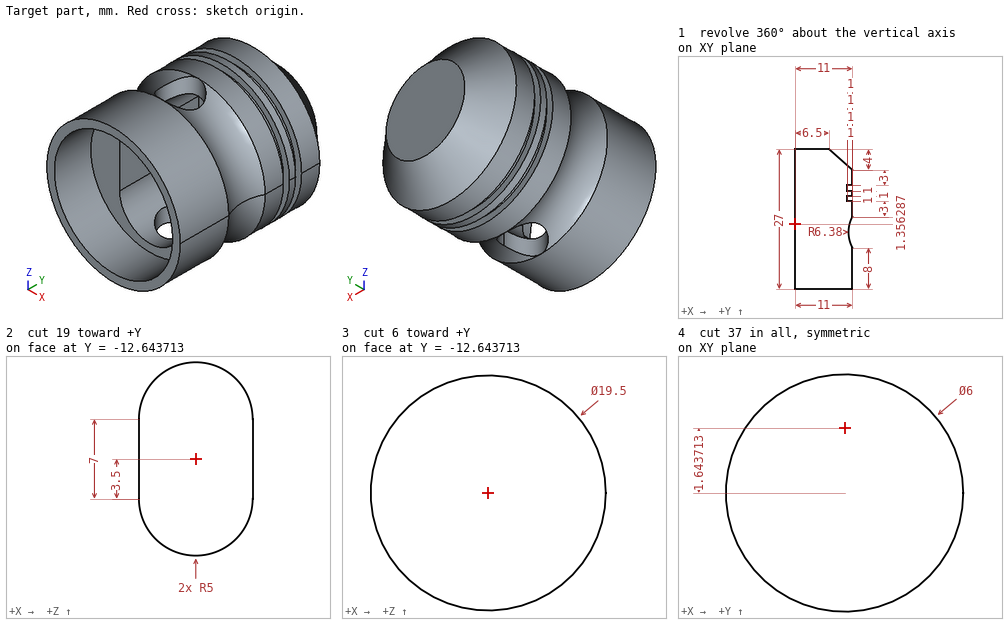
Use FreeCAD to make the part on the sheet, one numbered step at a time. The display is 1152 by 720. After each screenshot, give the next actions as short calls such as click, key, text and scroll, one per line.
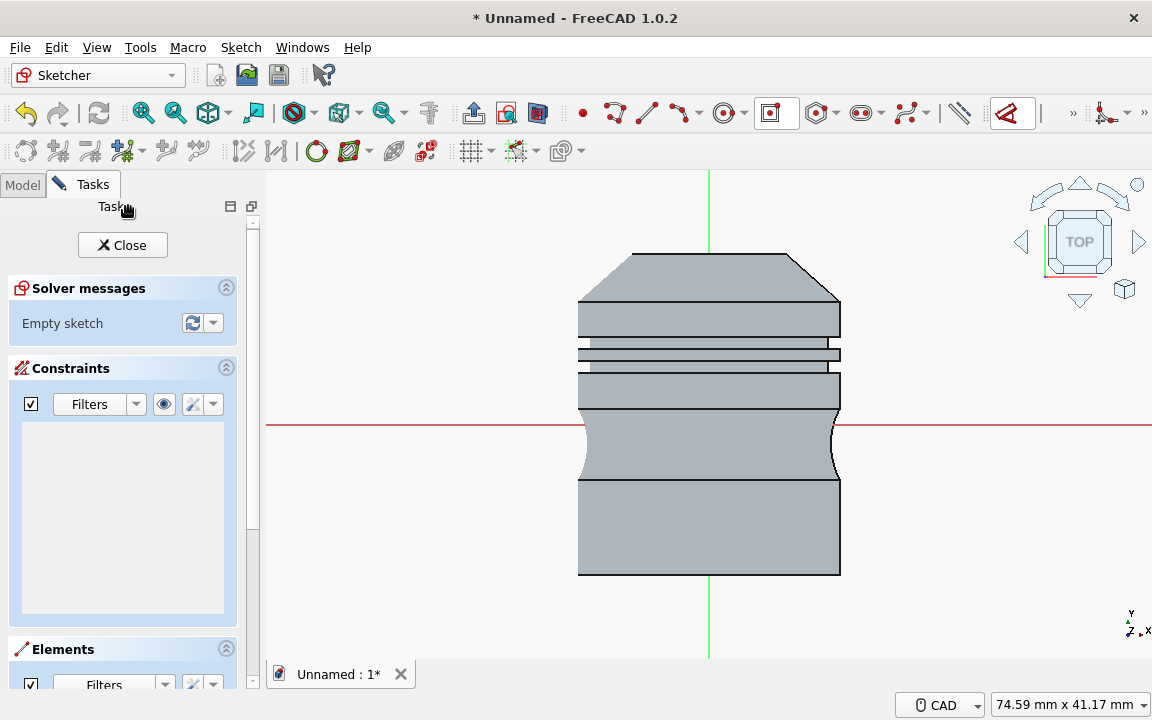
click(538, 114)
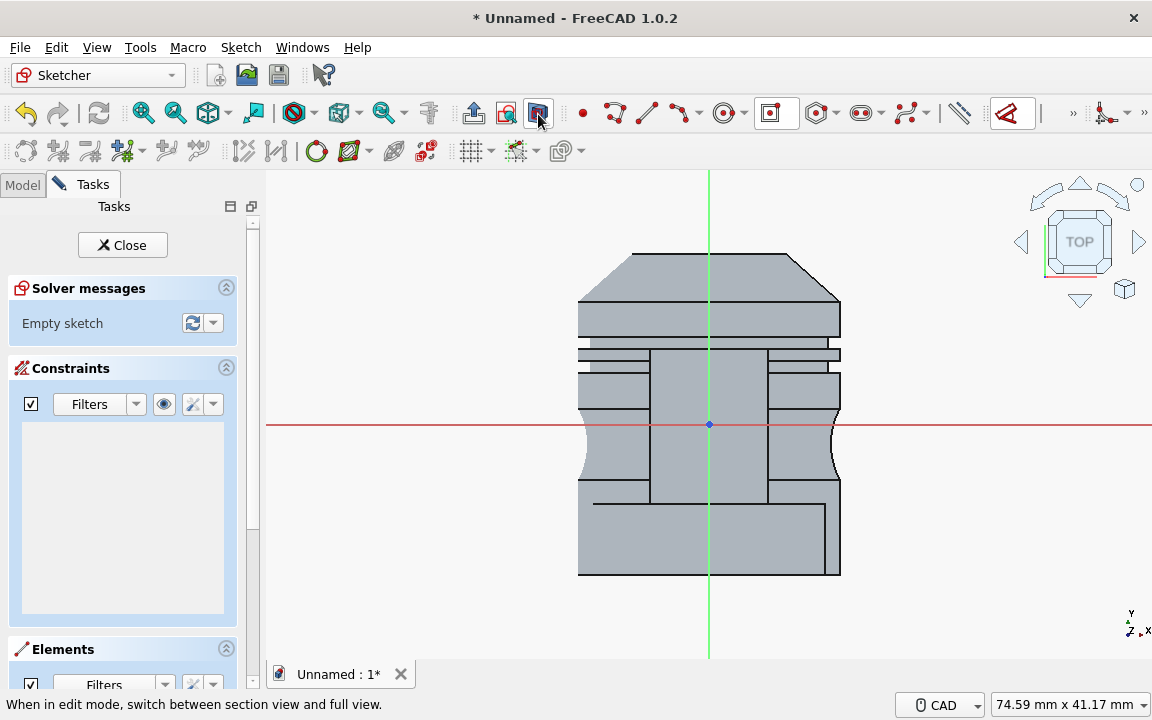
scroll(731, 454, up, 7)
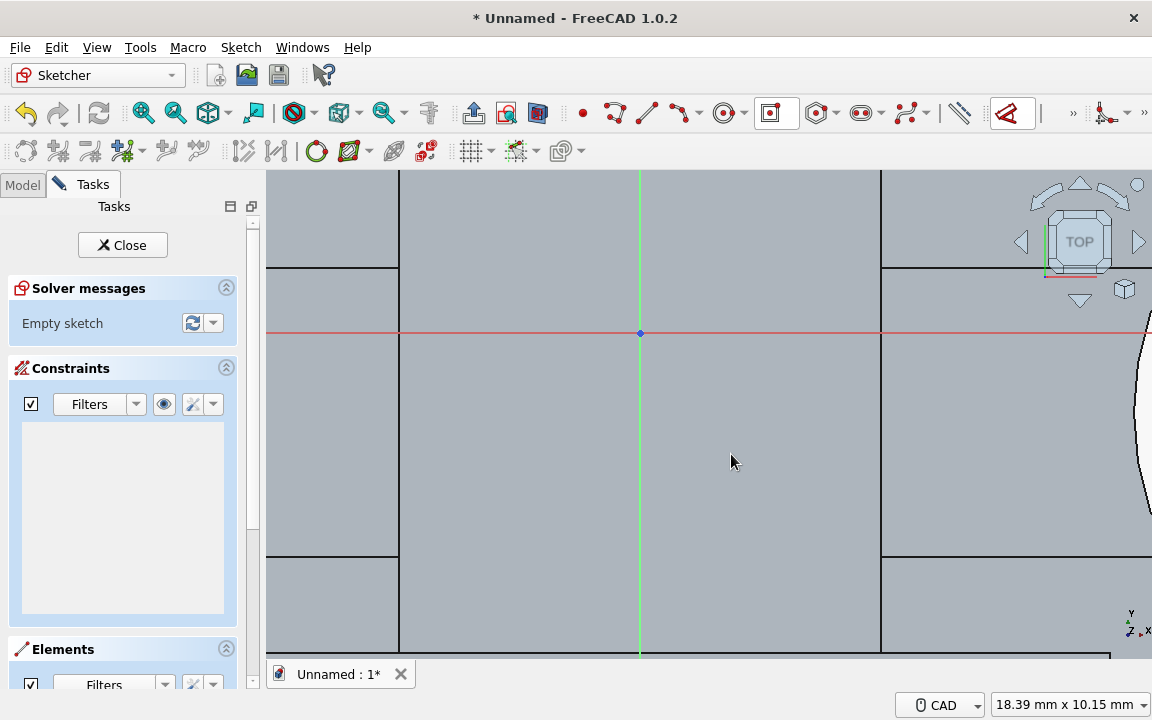
click(724, 114)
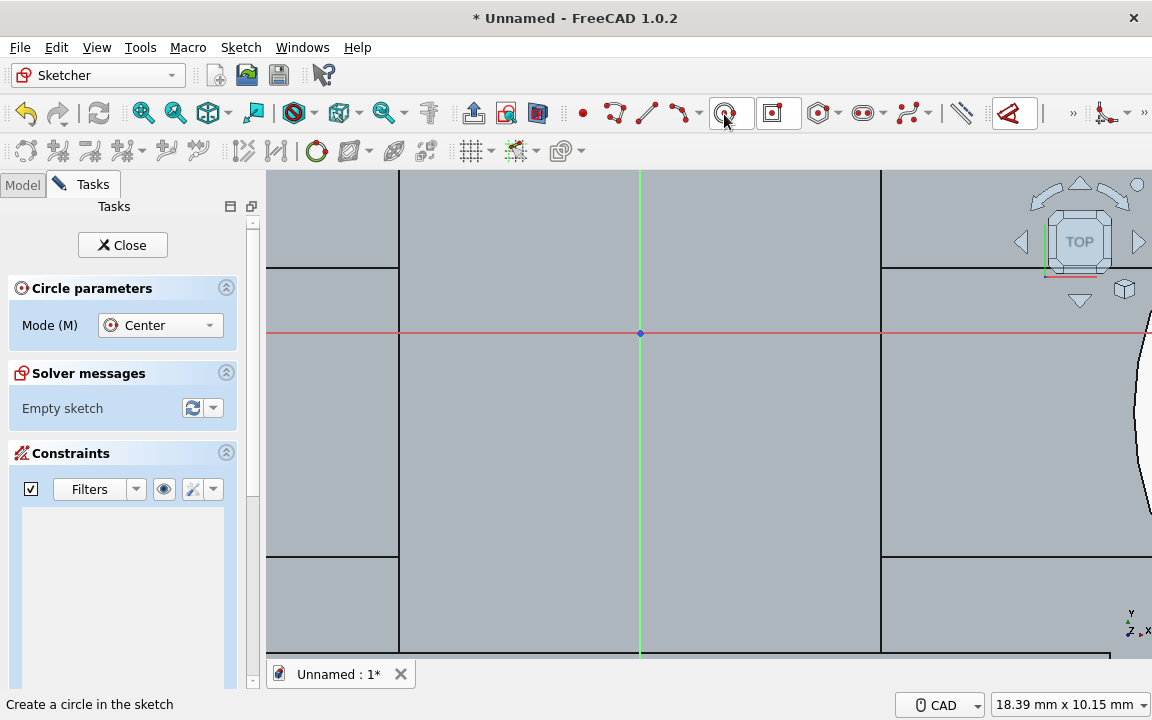
click(640, 412)
move(742, 310)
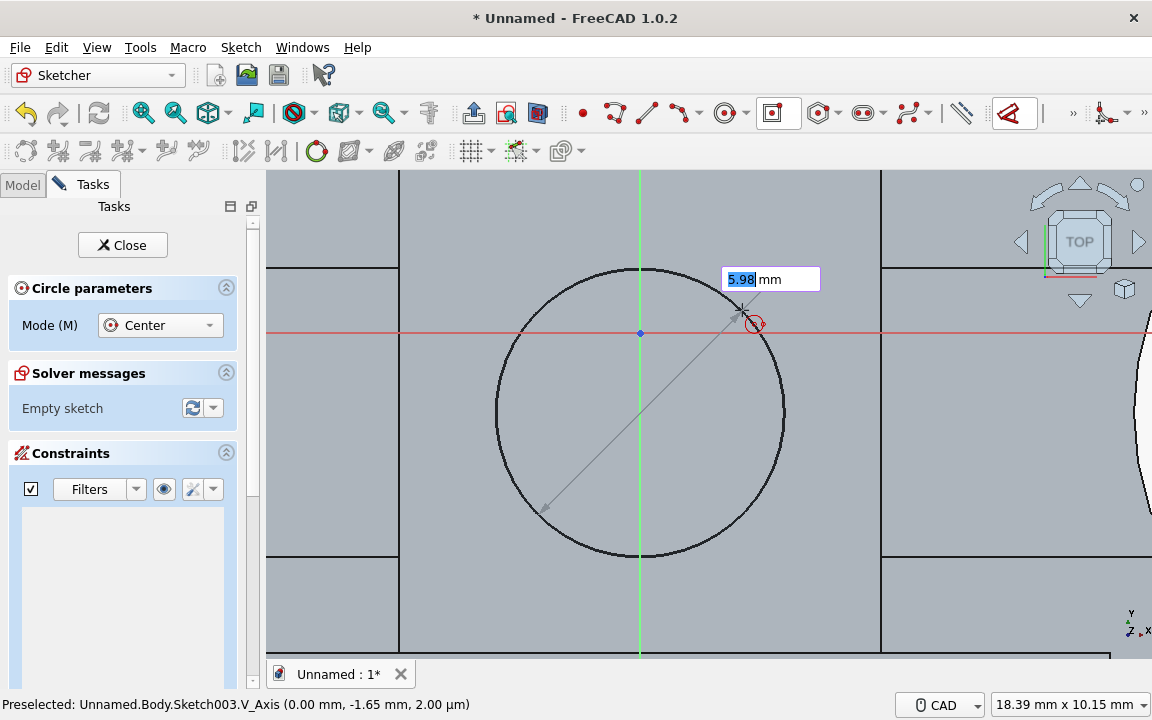
text(6)
key(Return)
key(Escape)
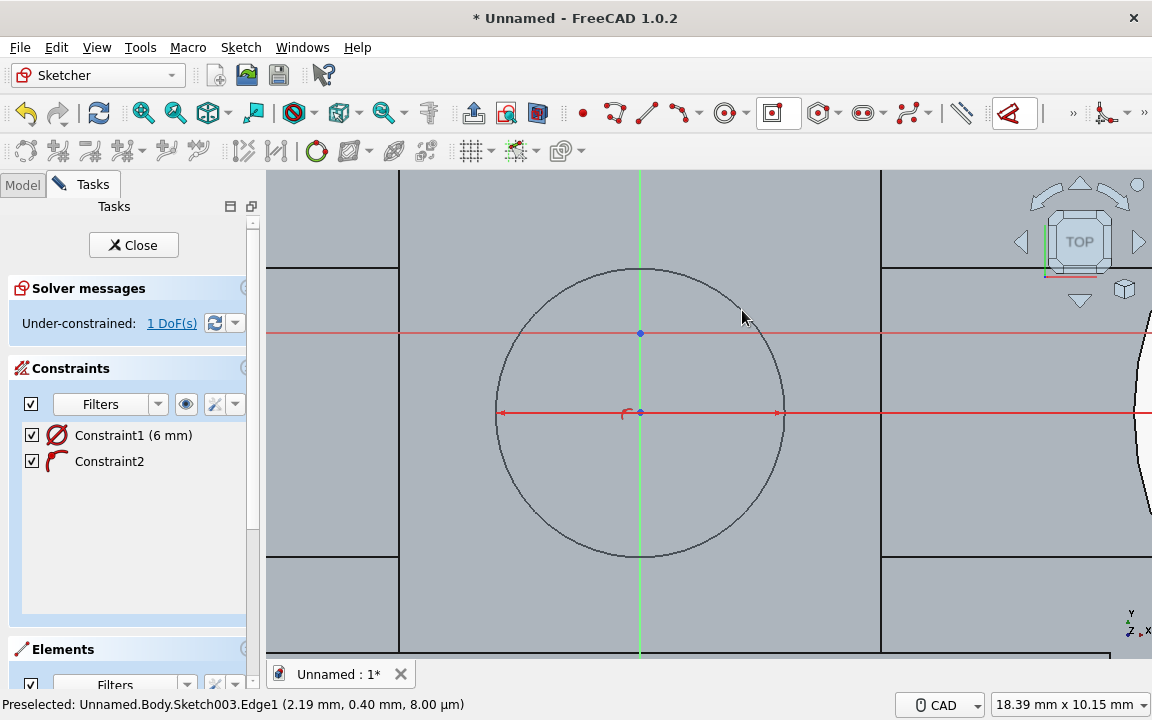
click(640, 413)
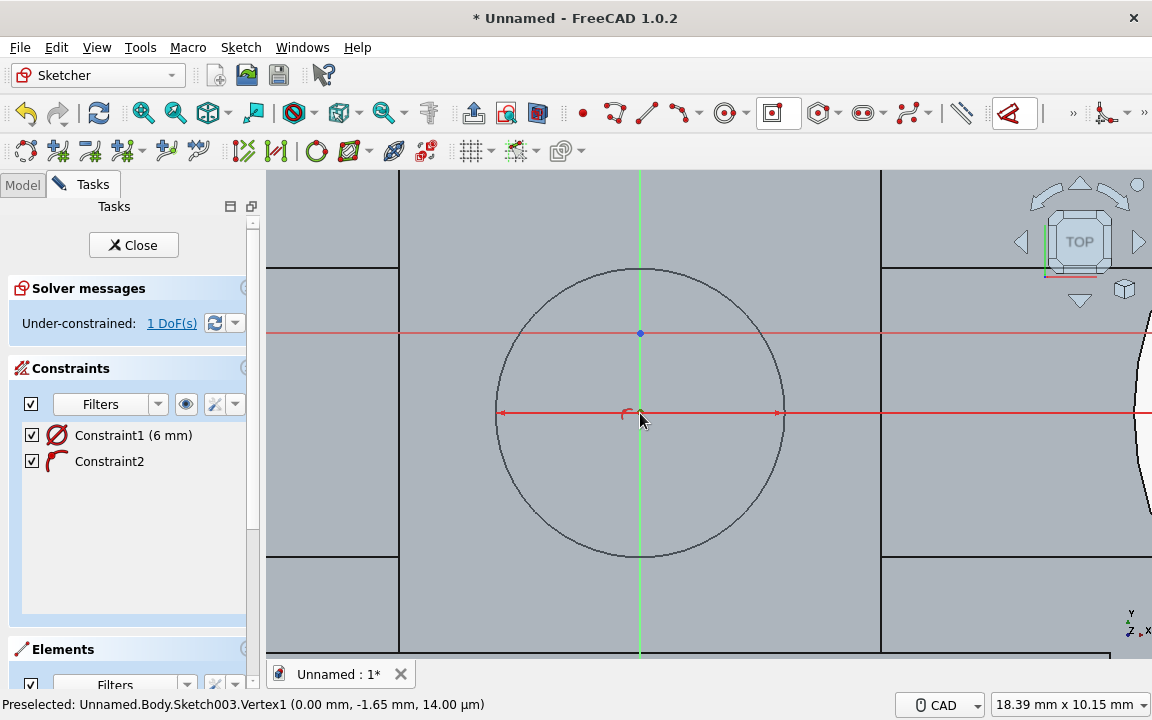
click(1032, 114)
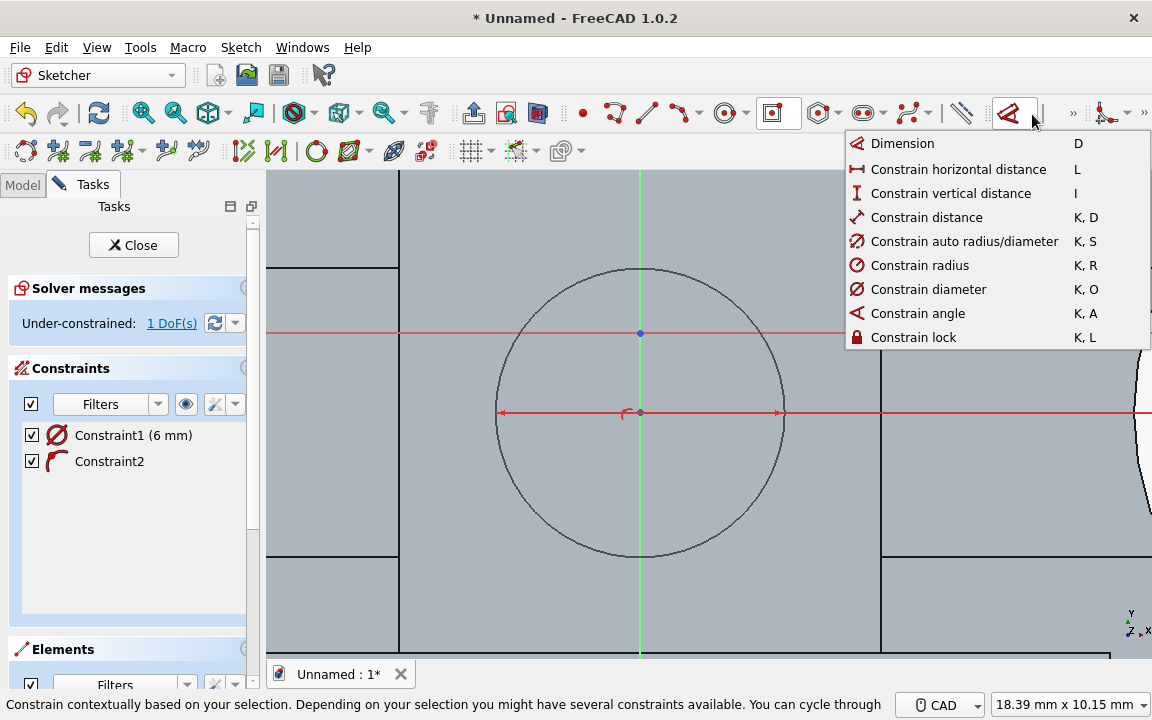
click(998, 193)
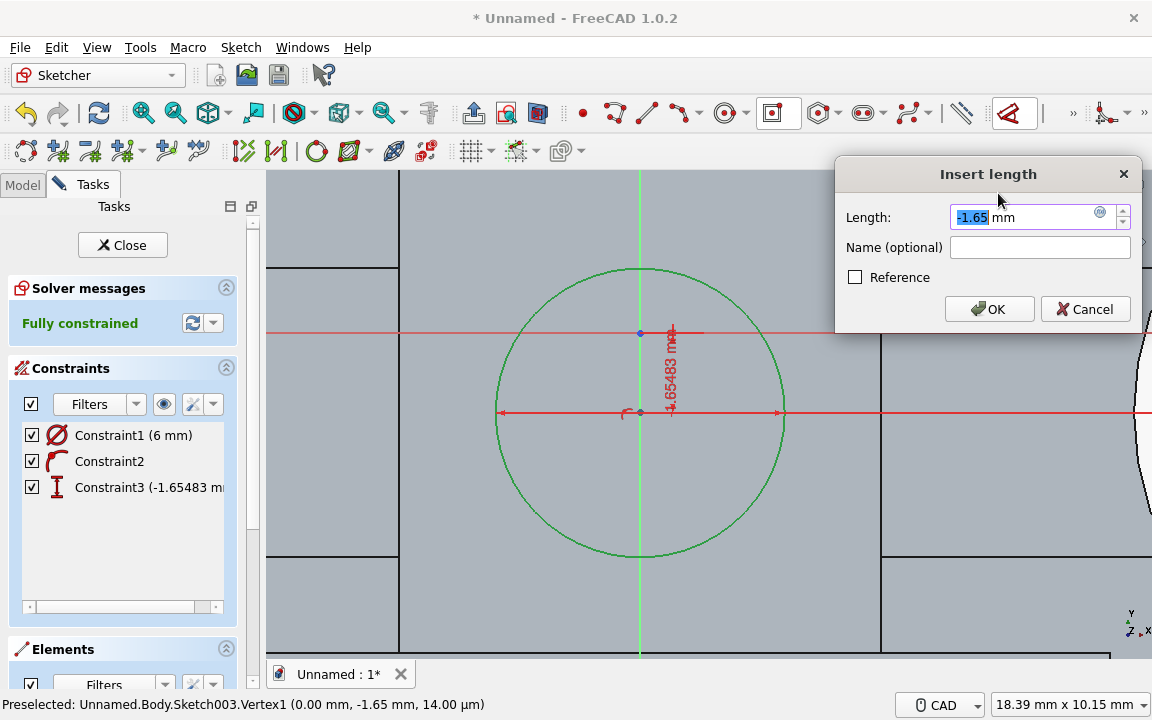
text(-1.643713)
key(Return)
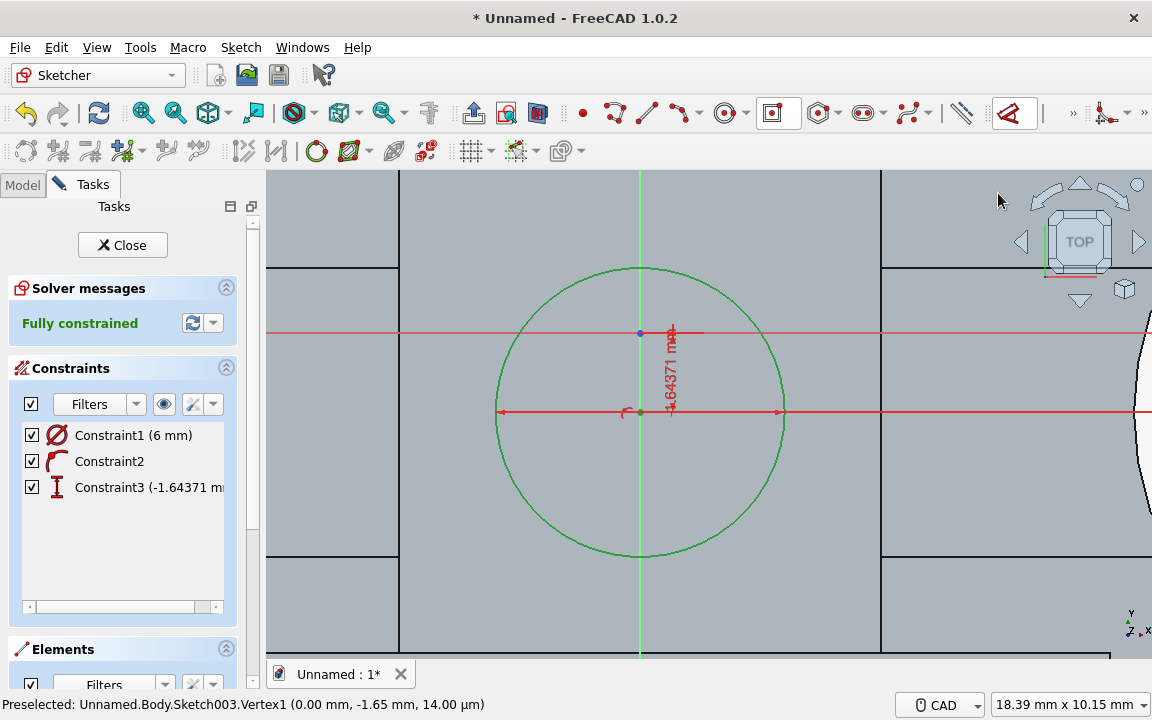
click(123, 245)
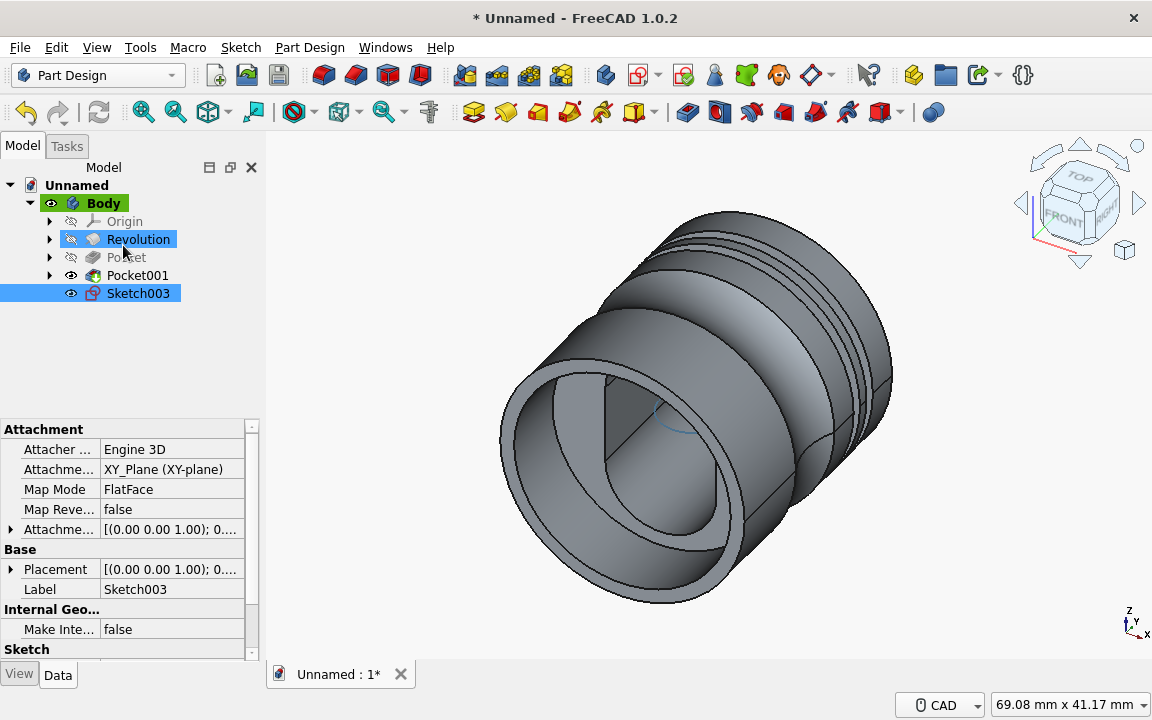
click(688, 112)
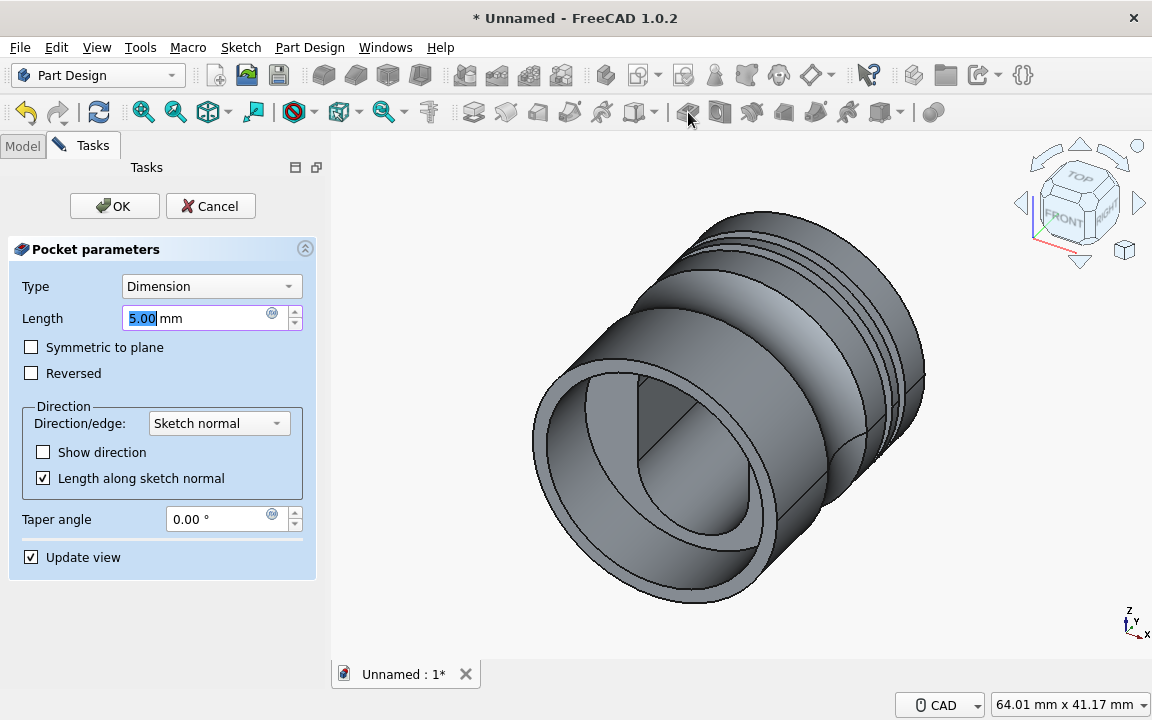
text(37)
key(Tab)